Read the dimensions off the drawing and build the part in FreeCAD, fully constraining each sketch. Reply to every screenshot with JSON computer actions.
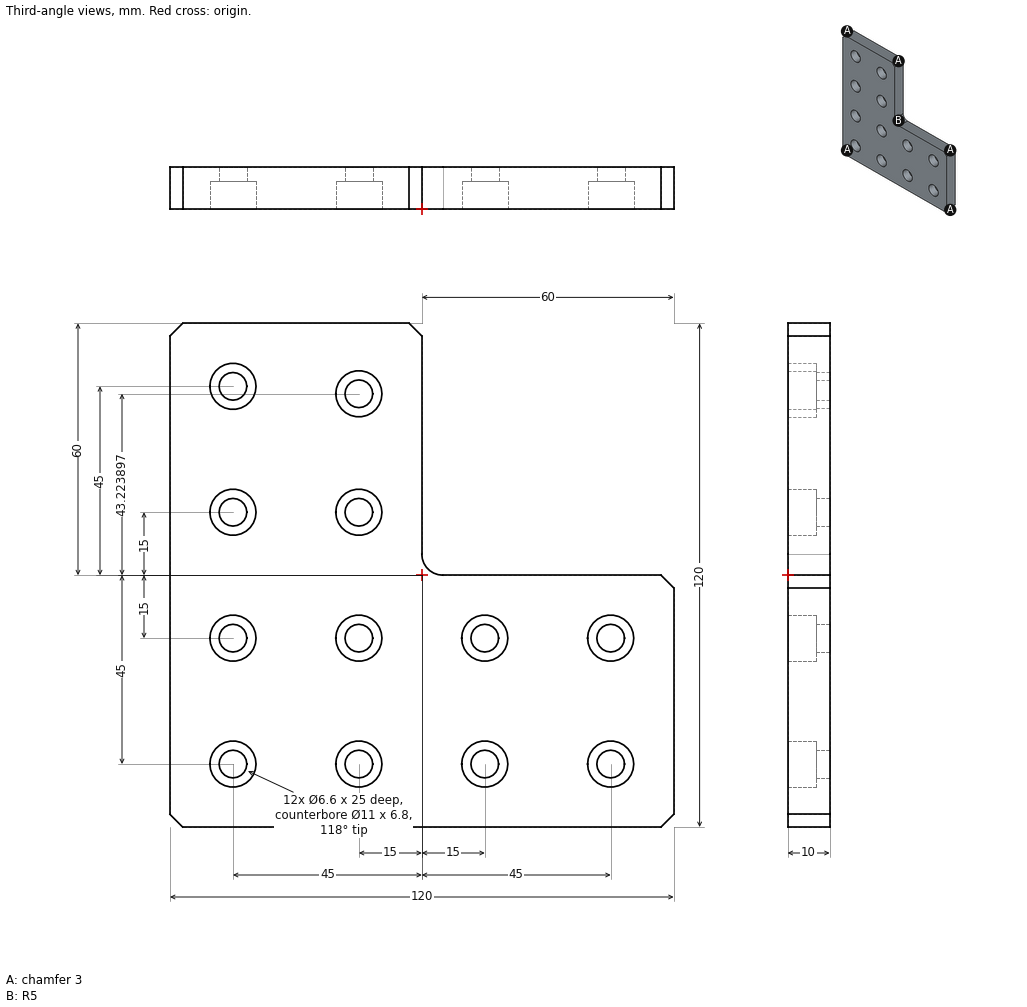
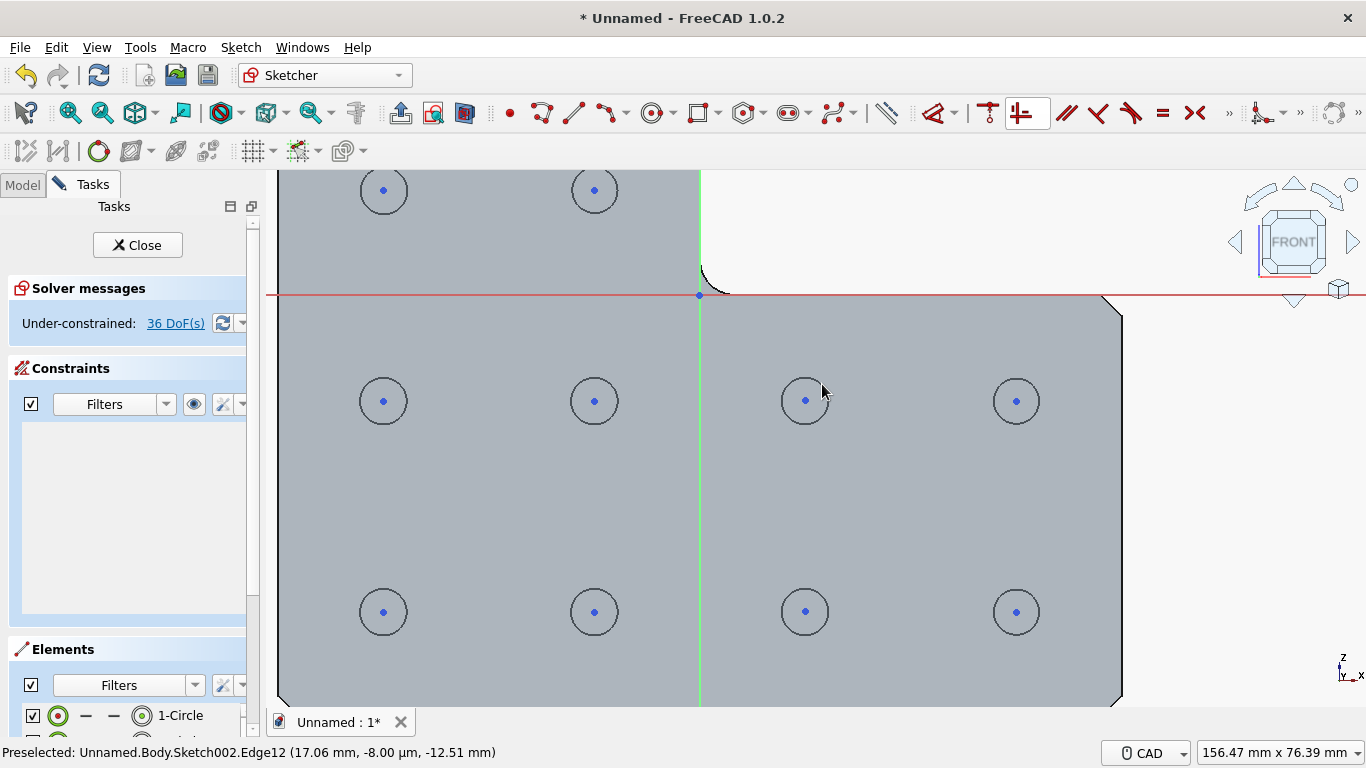
{"action": "left_click", "coordinate": [400, 596]}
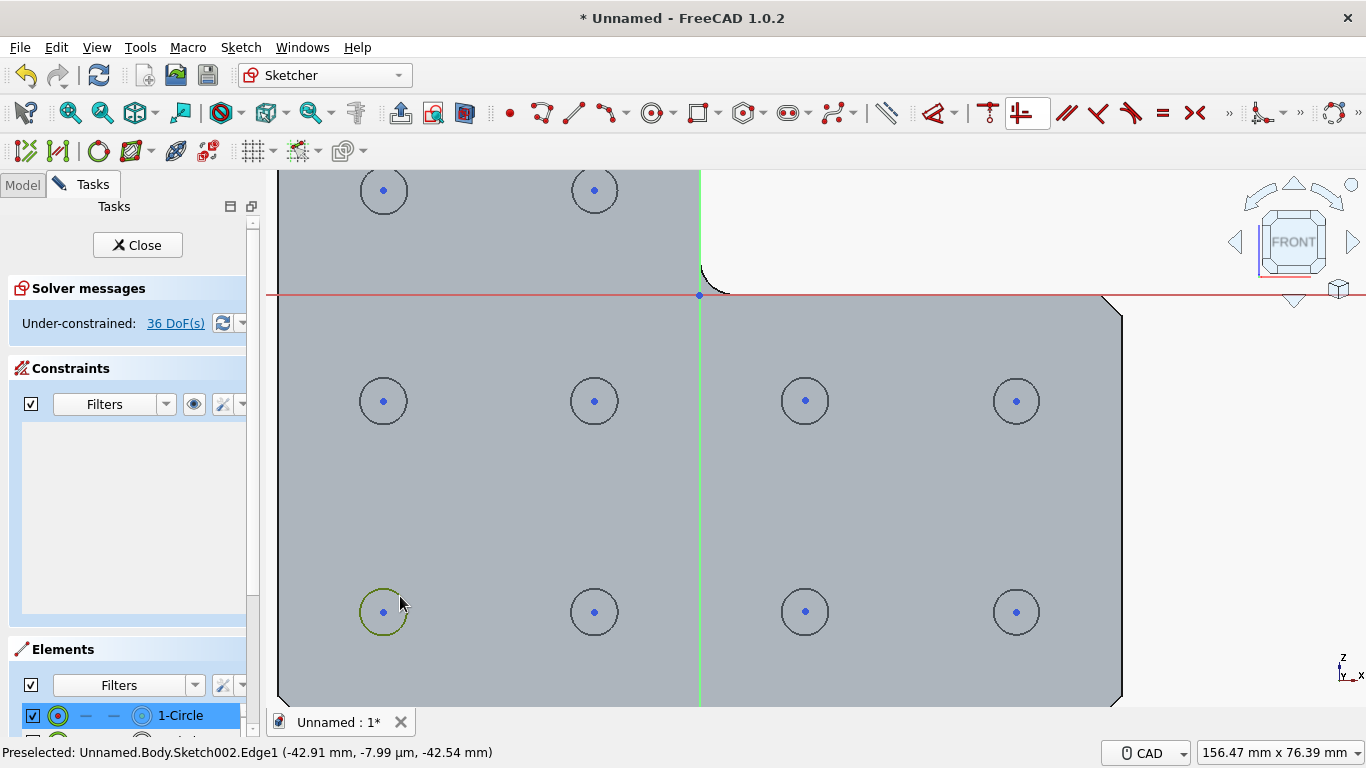
{"action": "left_click", "coordinate": [400, 385]}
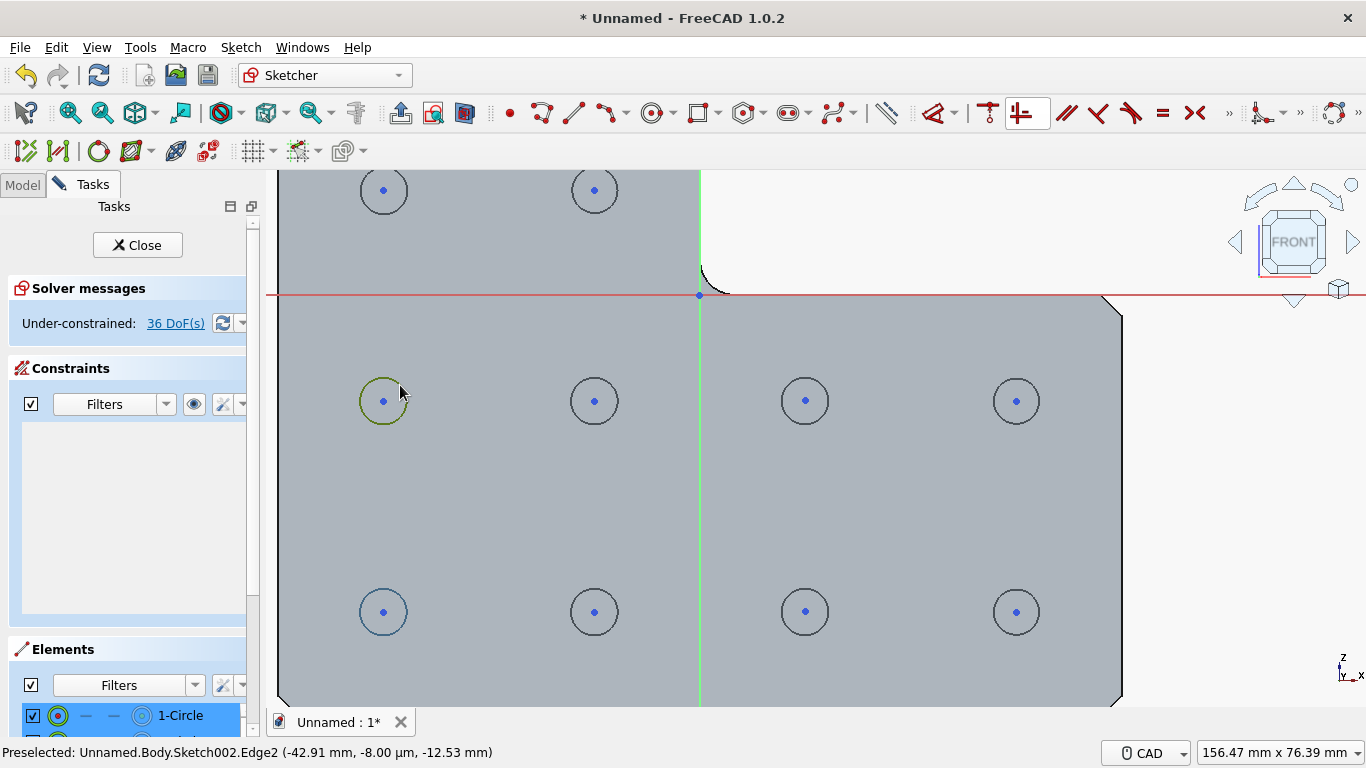
{"action": "left_click", "coordinate": [611, 596]}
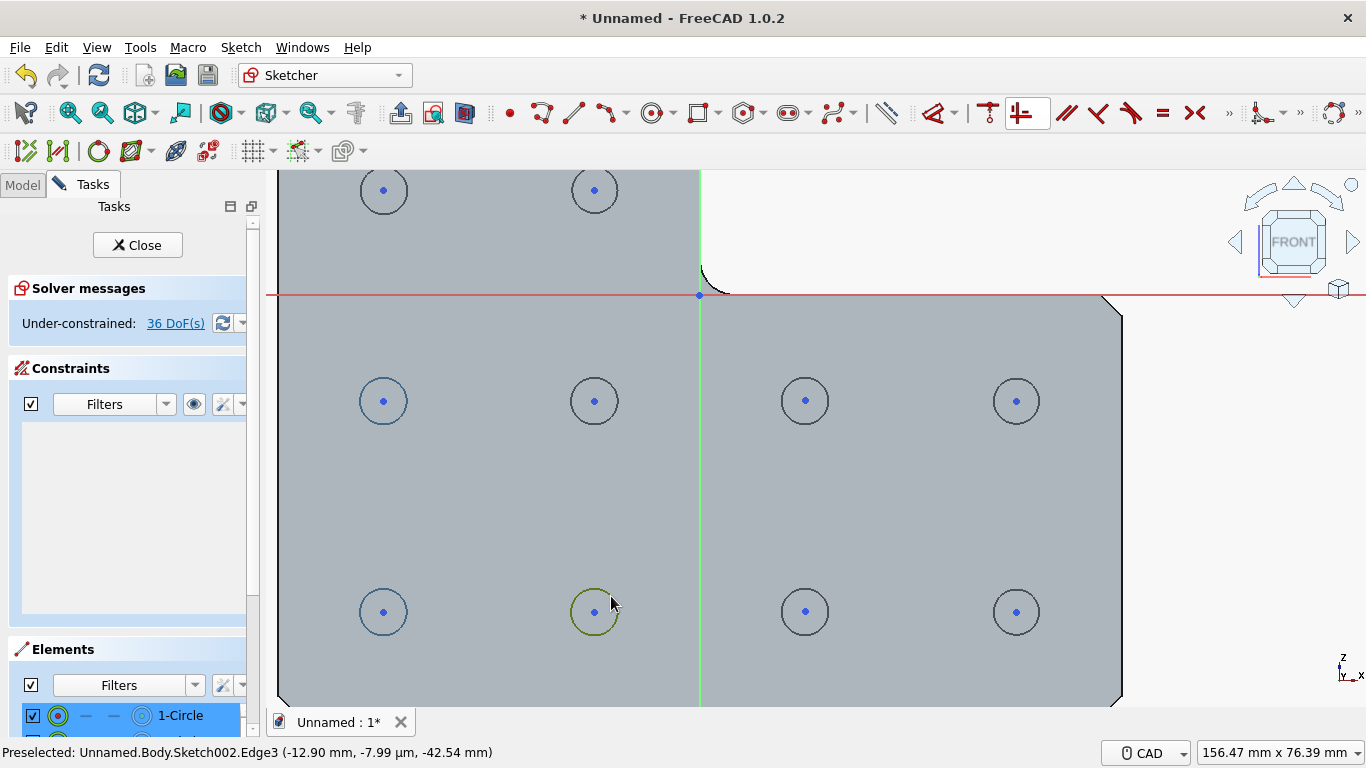
{"action": "left_click", "coordinate": [611, 385]}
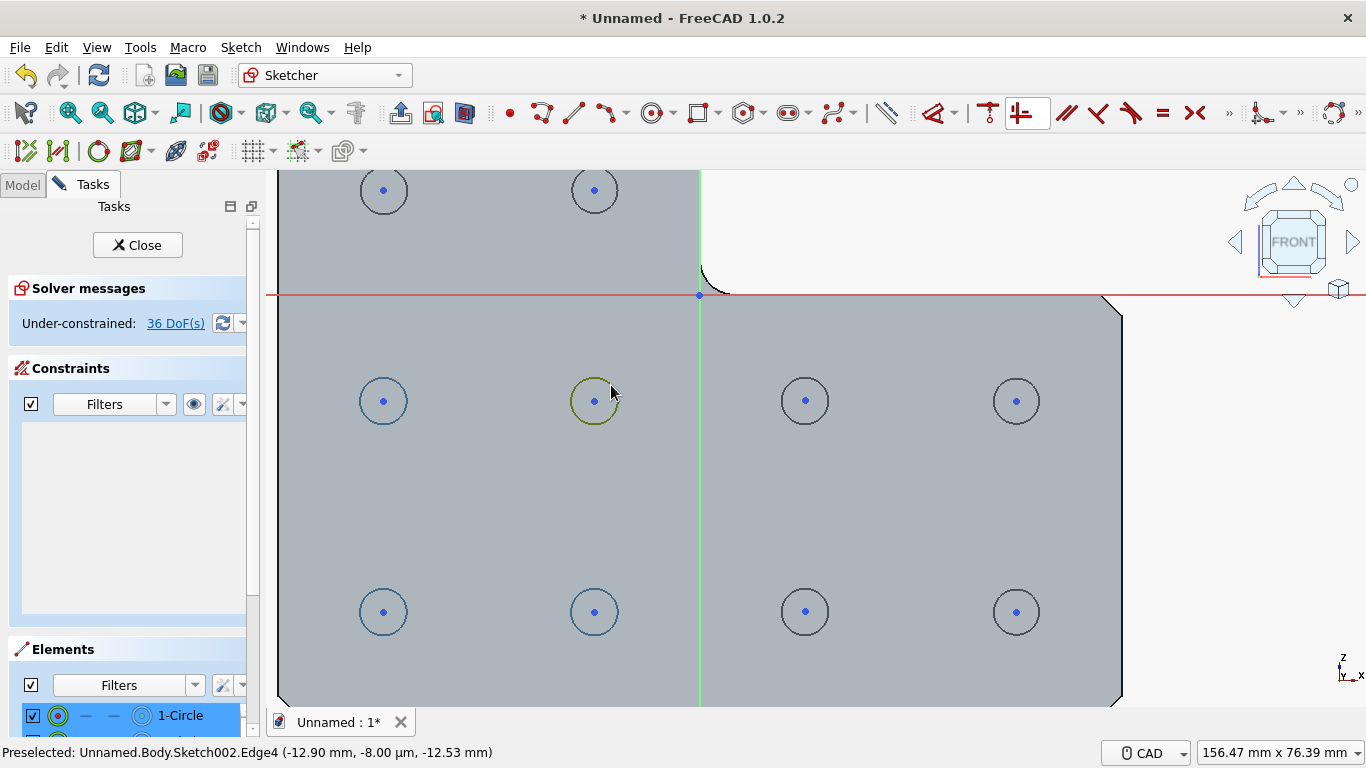
{"action": "left_click", "coordinate": [1032, 596]}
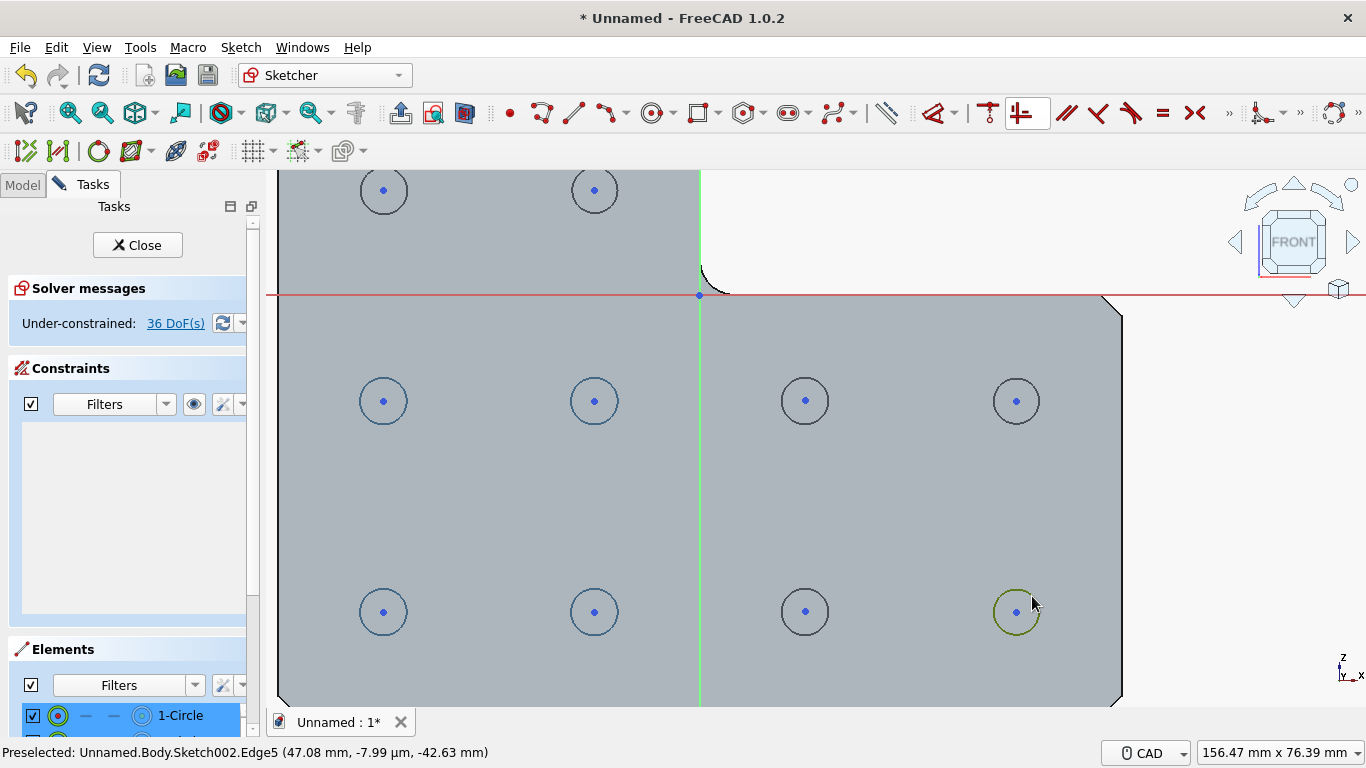
{"action": "left_click", "coordinate": [1032, 385]}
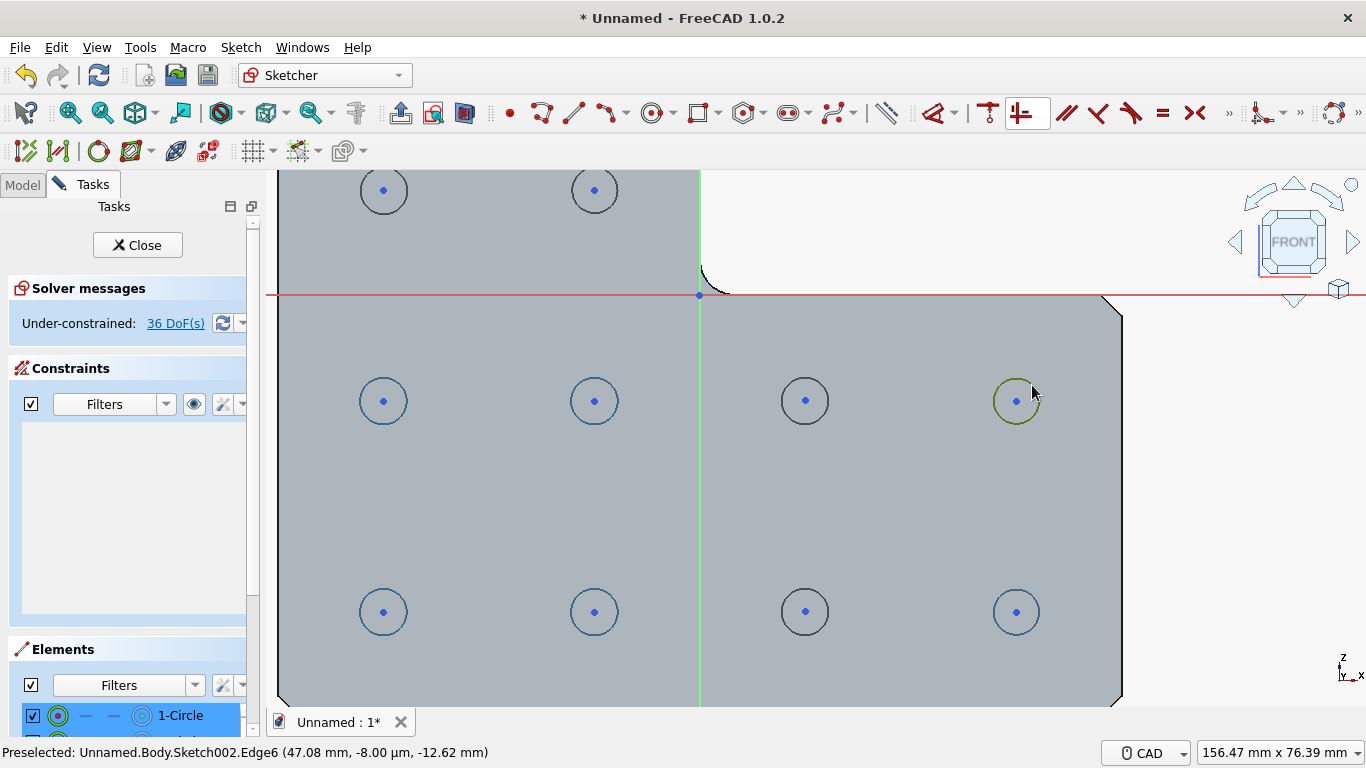
{"action": "left_click", "coordinate": [367, 207]}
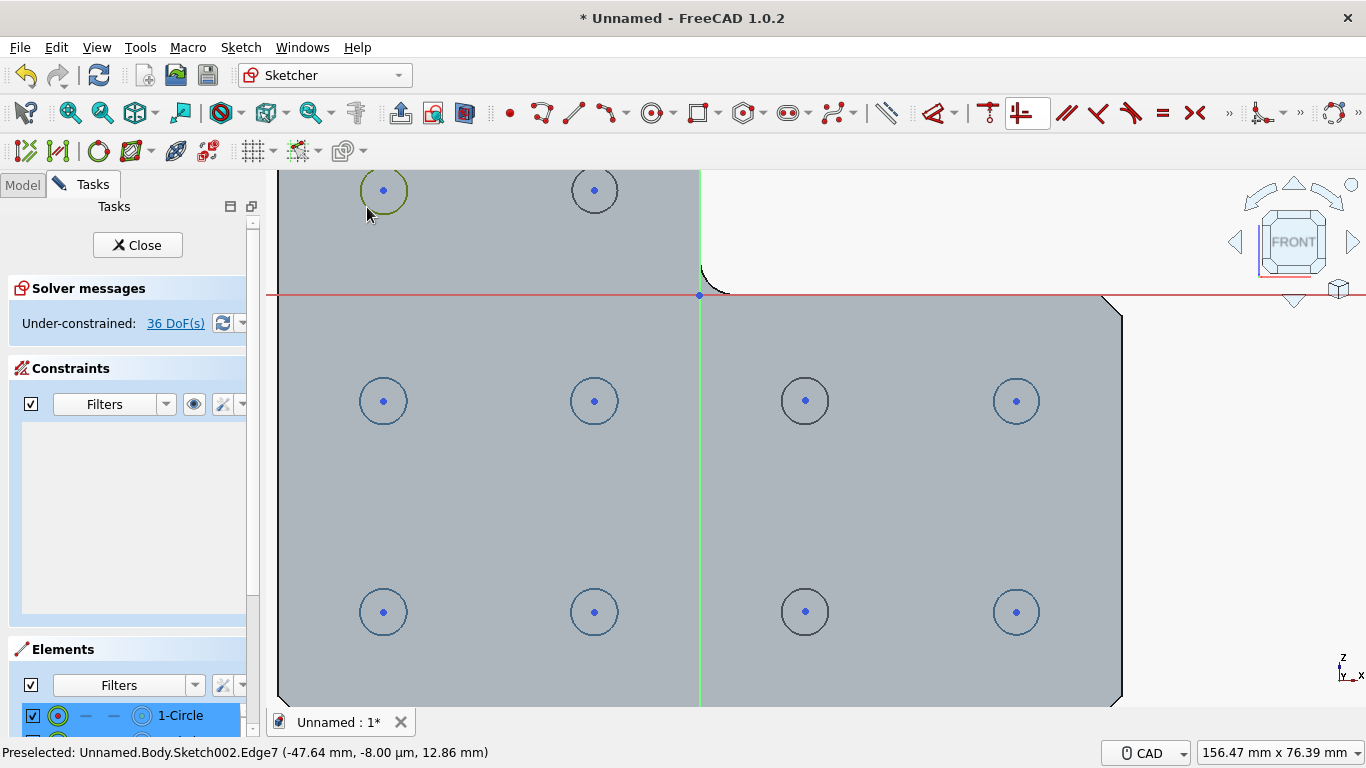
{"action": "scroll", "coordinate": [805, 613], "scroll_direction": "down", "scroll_amount": 3}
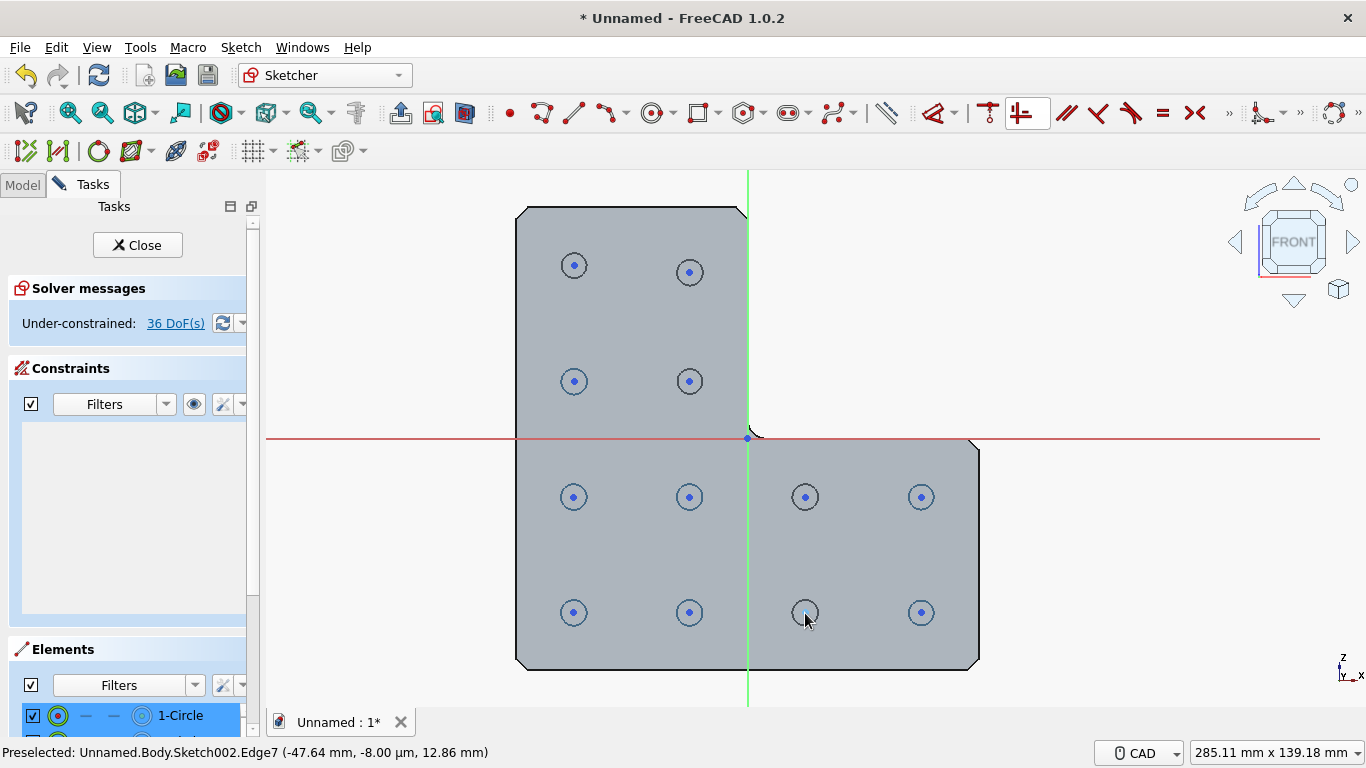
{"action": "left_click", "coordinate": [583, 257]}